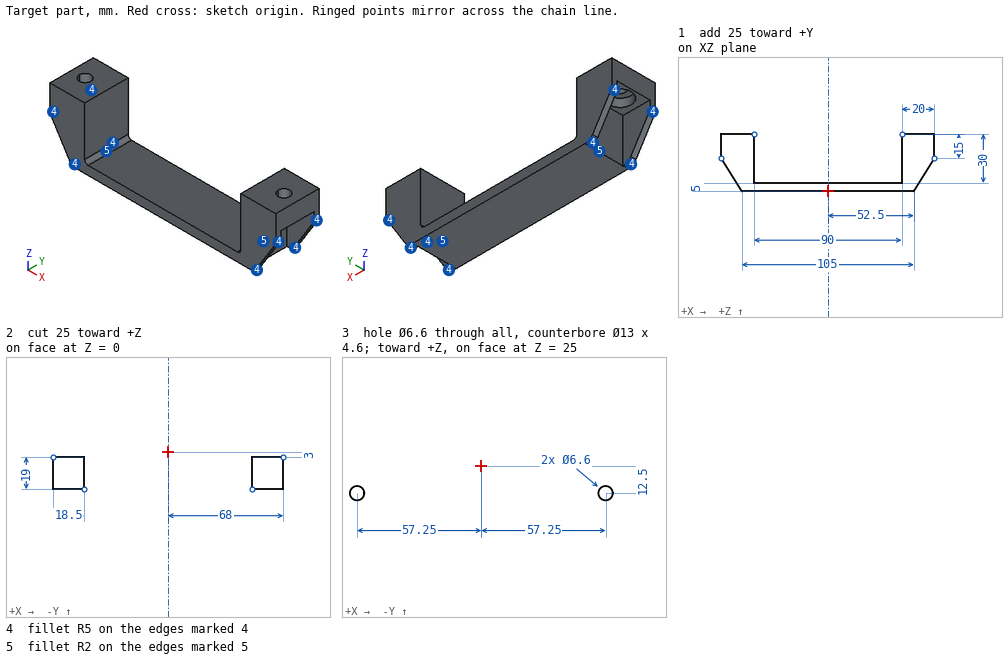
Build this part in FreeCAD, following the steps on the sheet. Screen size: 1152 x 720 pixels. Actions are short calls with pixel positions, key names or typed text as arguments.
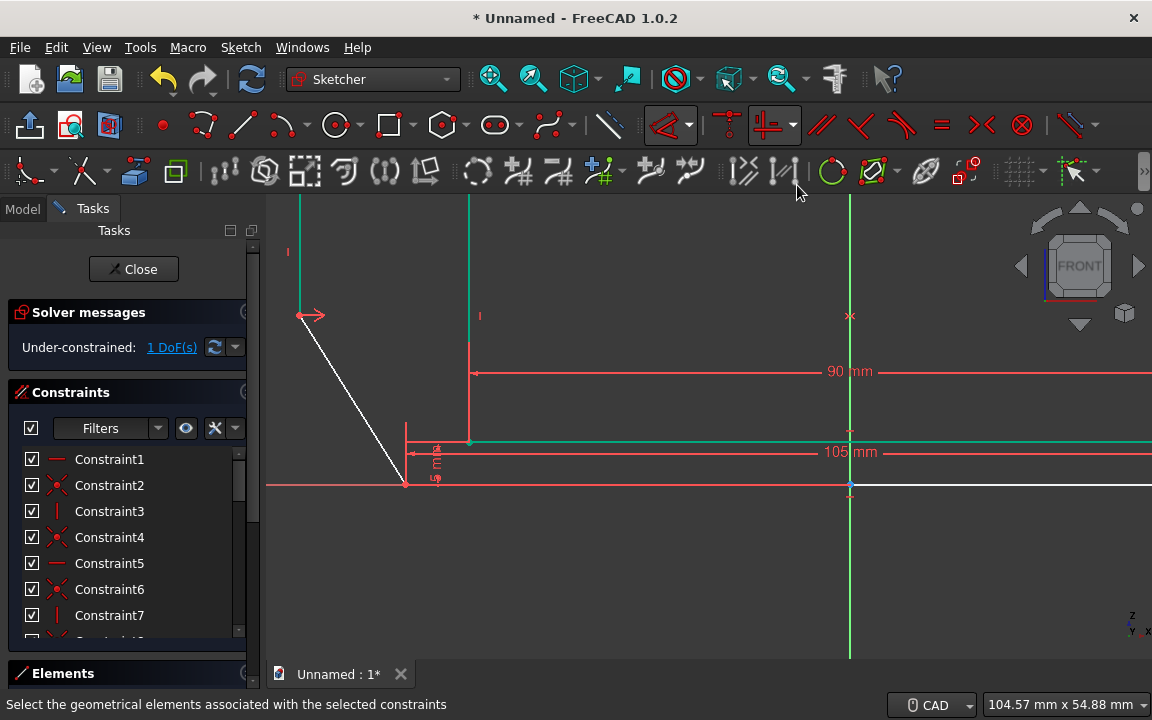
scroll(469, 500, down, 4)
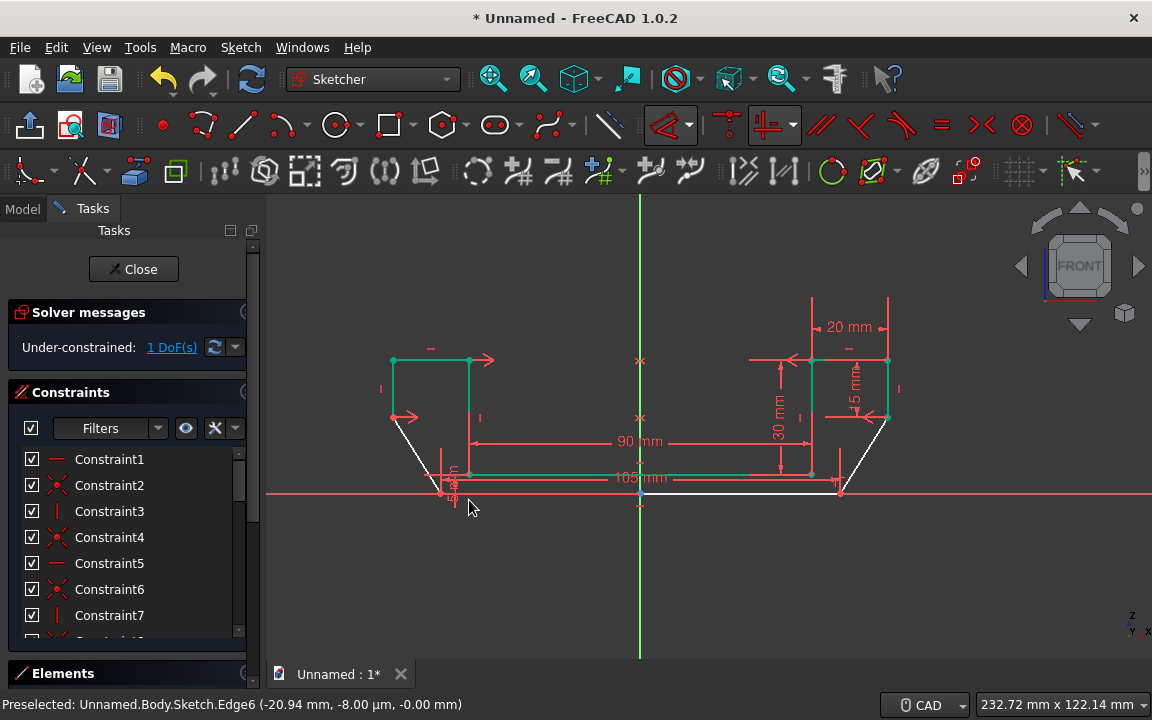
click(840, 494)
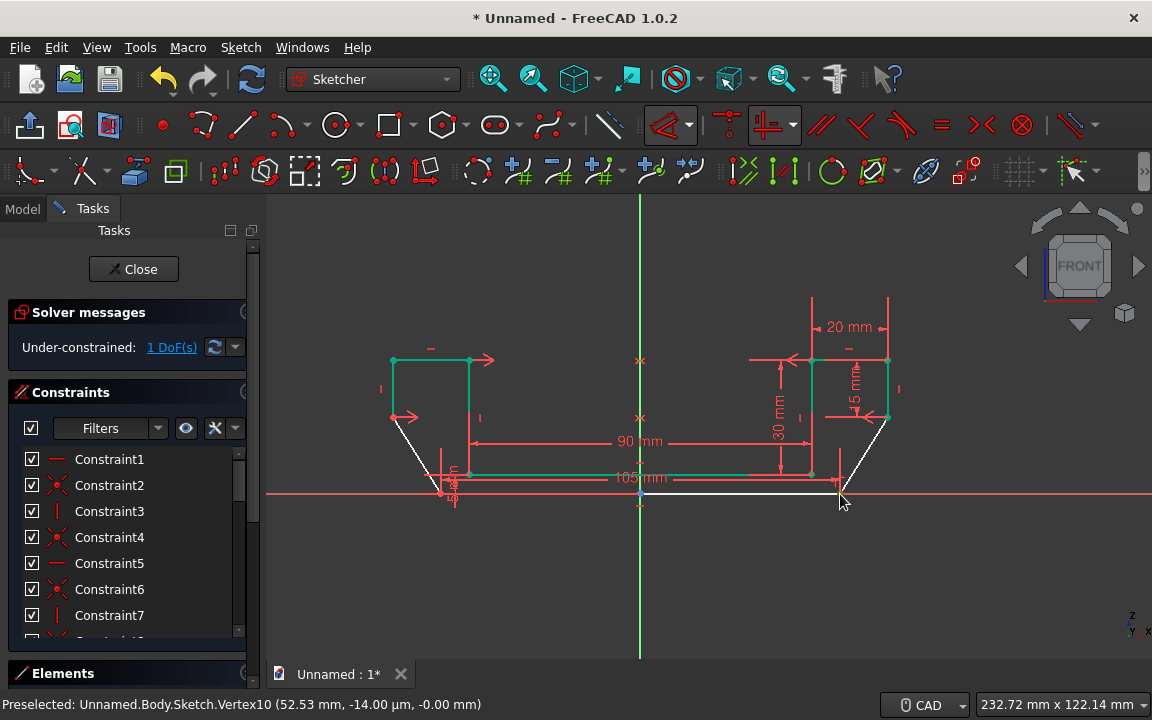
key(l)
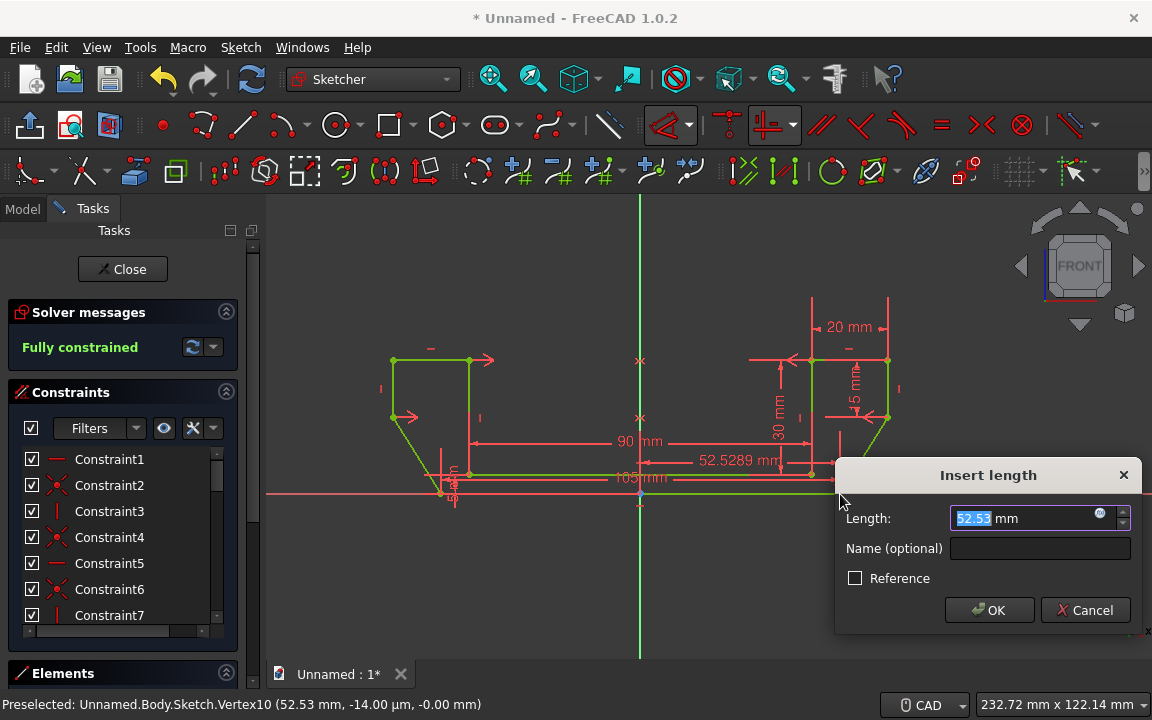
text(52.5)
key(Return)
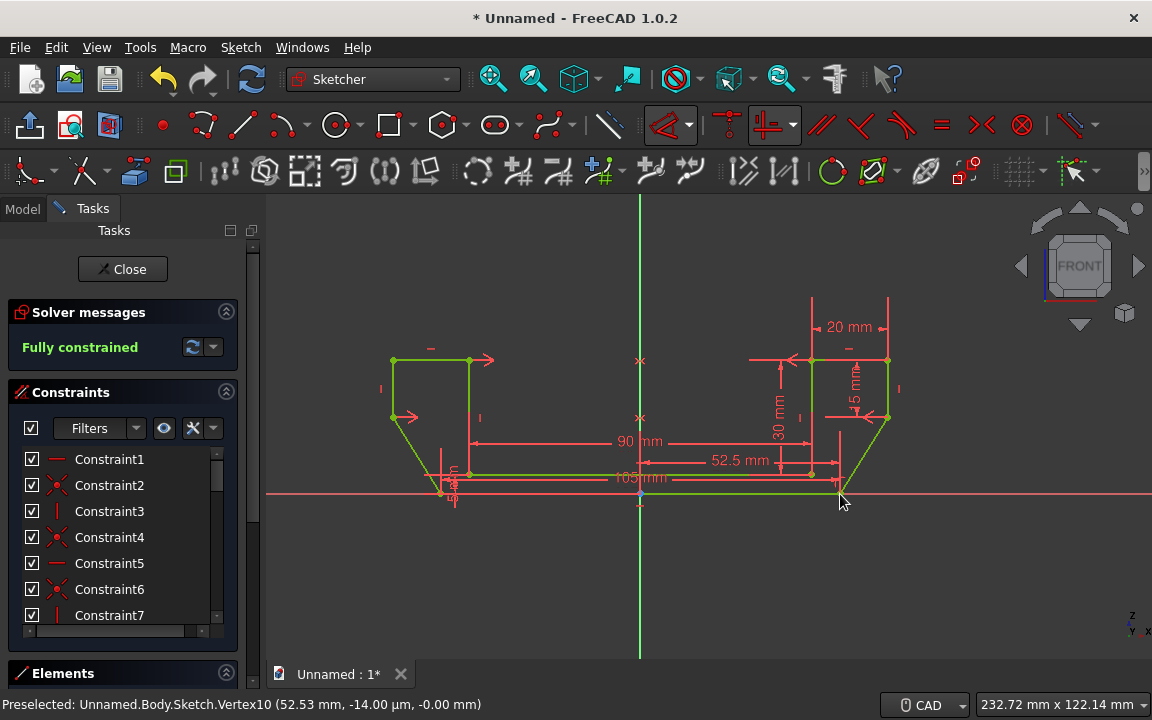
click(123, 269)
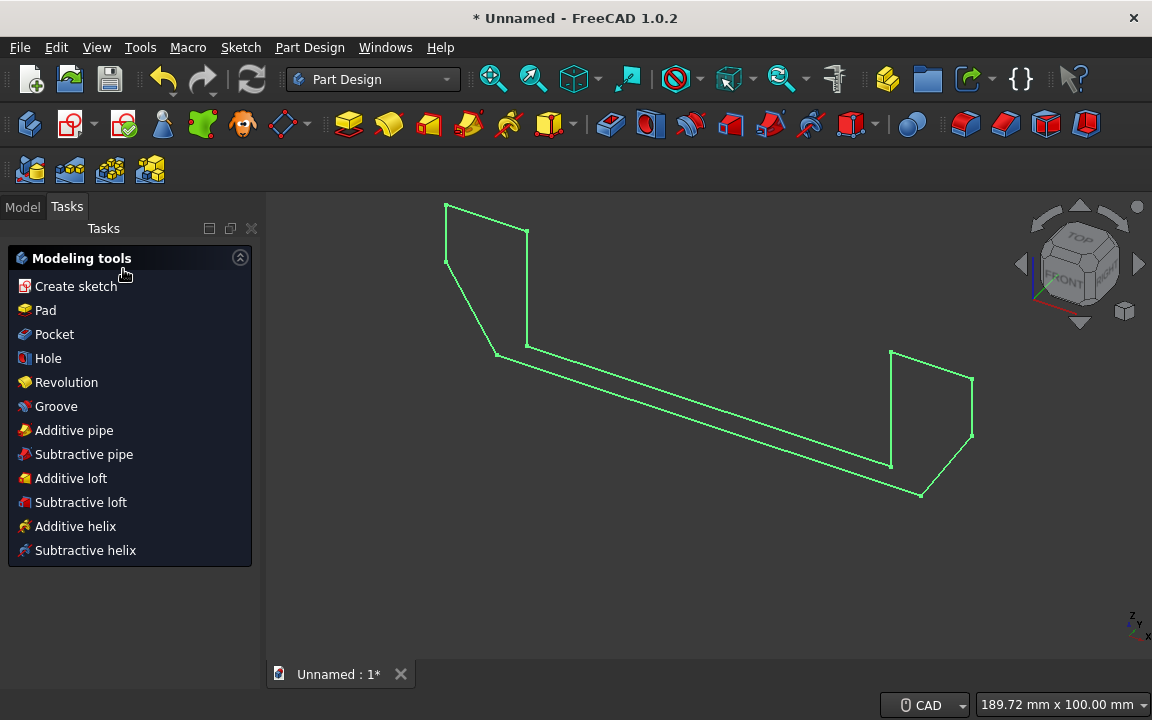
click(350, 124)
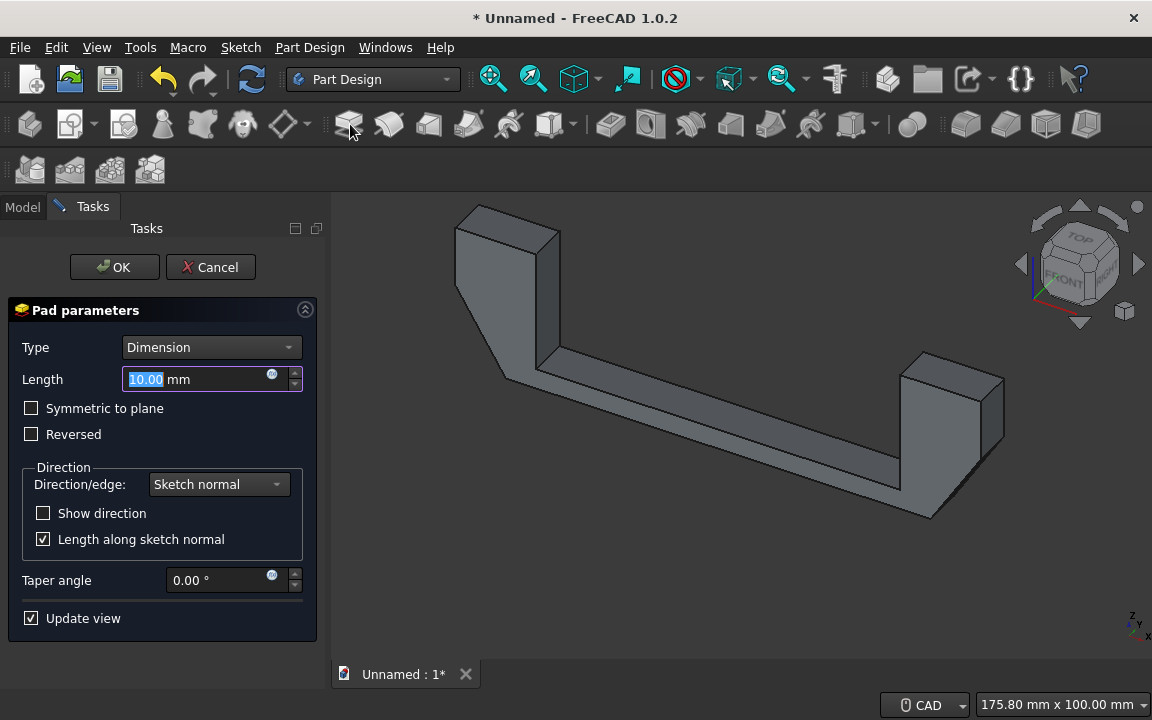
text(25)
key(Tab)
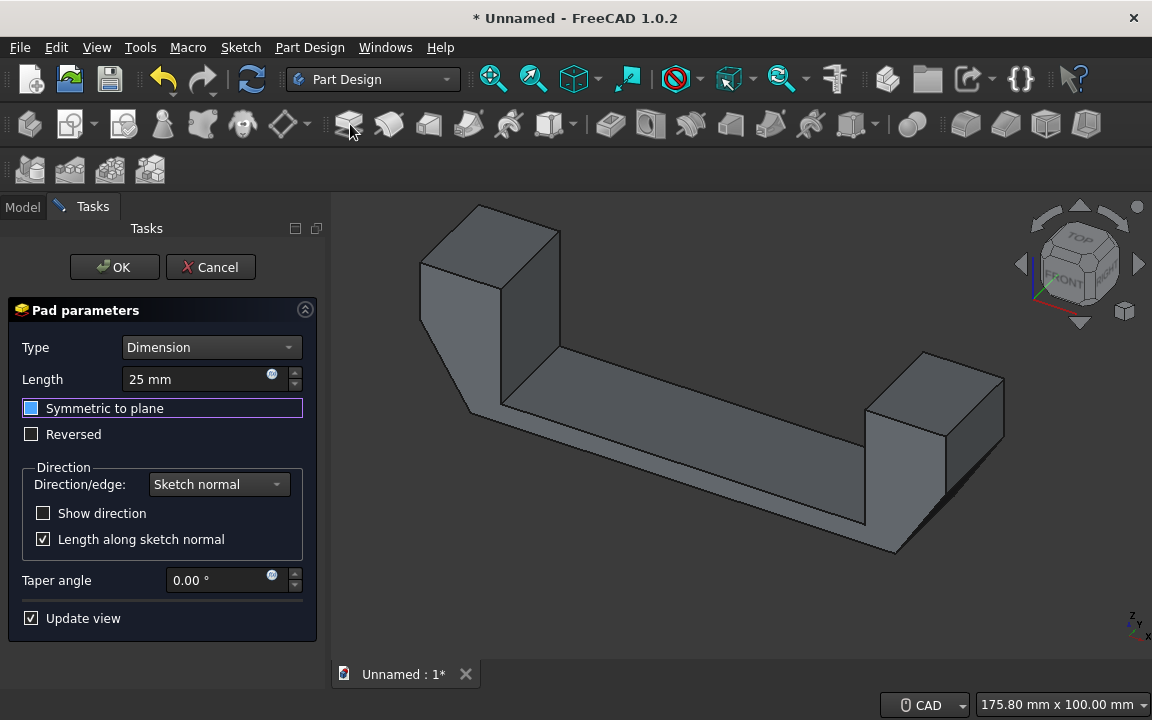
click(30, 434)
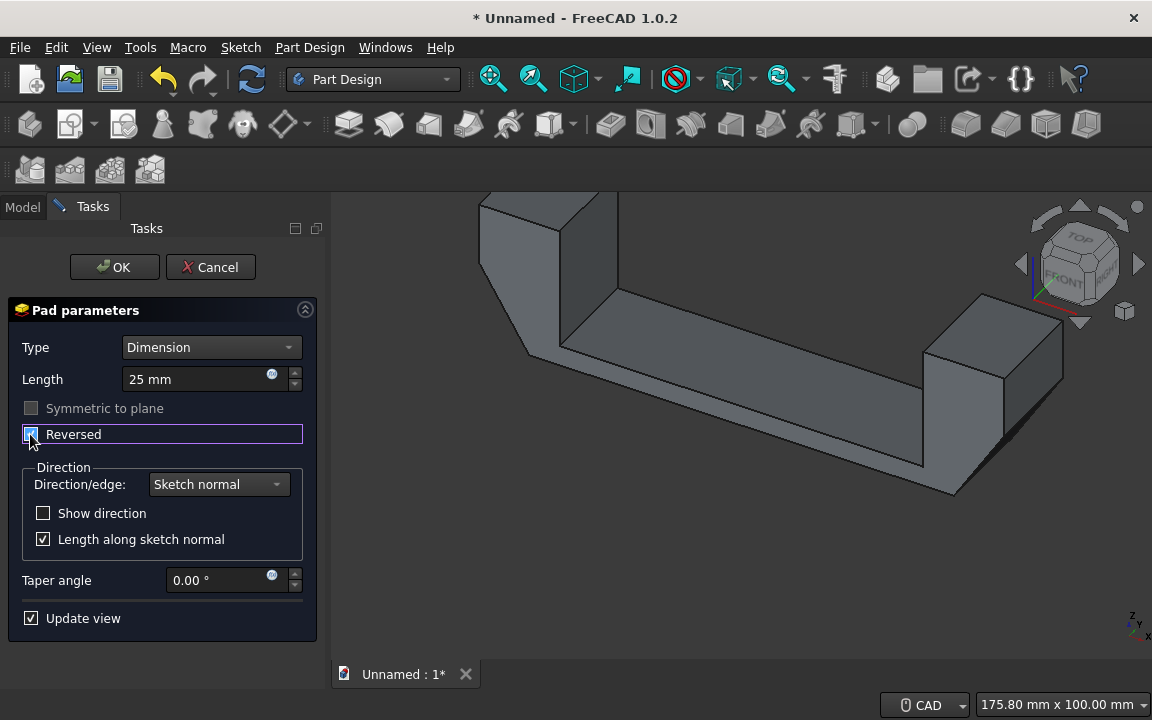
click(115, 267)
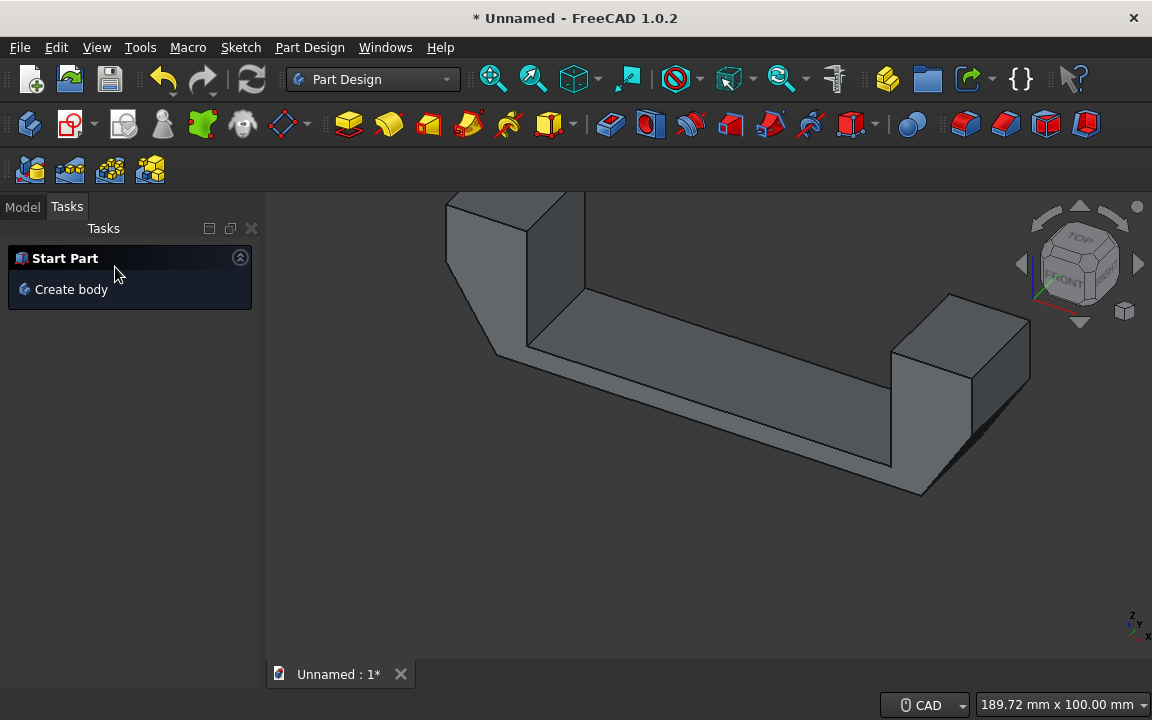
click(494, 80)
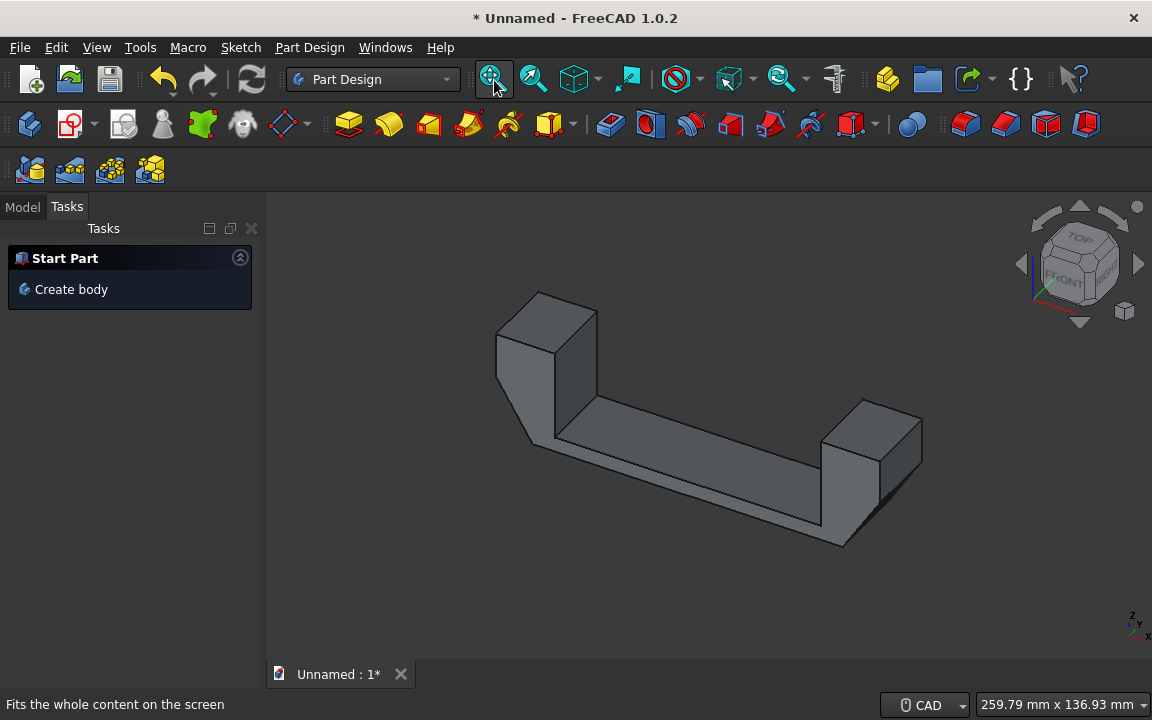
key(5)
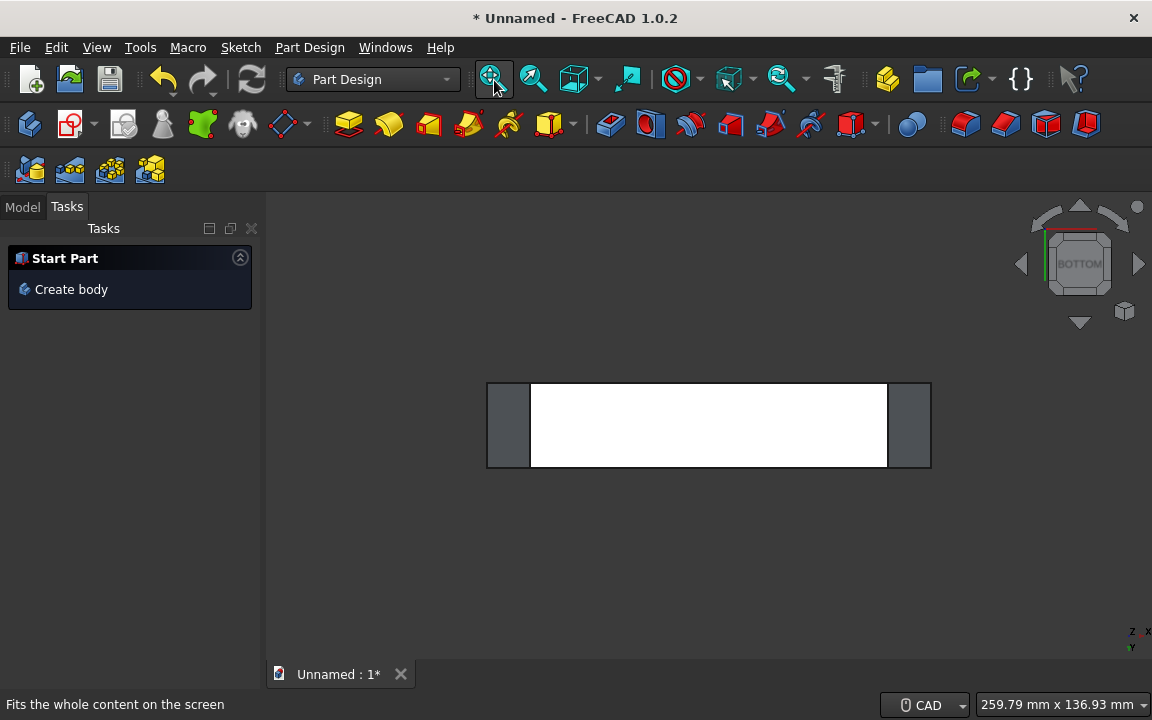
click(811, 424)